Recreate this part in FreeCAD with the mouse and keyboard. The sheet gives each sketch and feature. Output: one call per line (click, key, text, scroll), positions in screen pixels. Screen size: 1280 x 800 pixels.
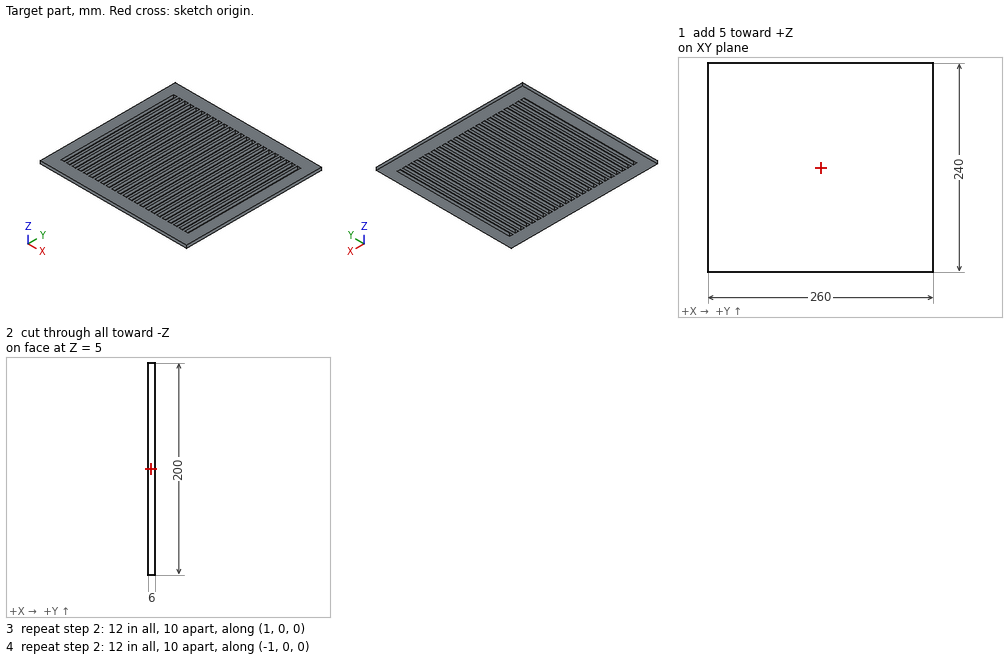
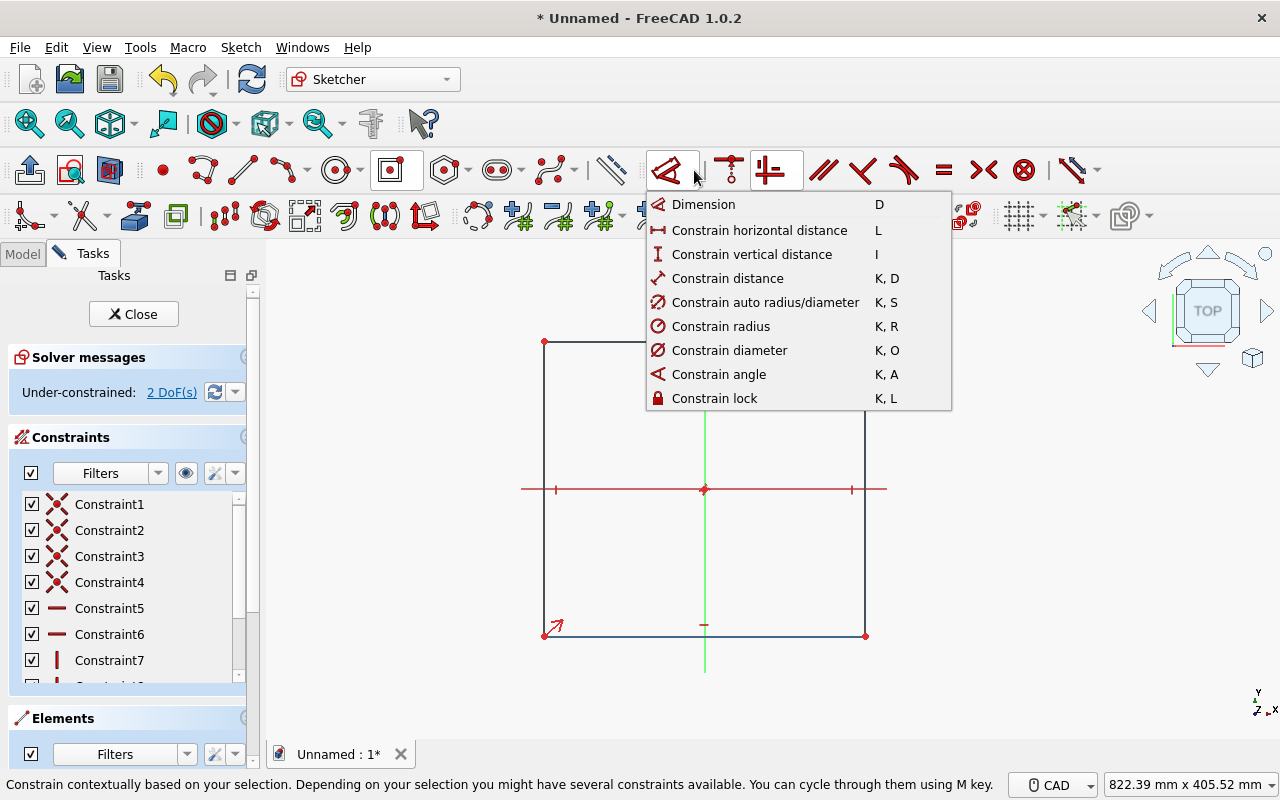
click(799, 230)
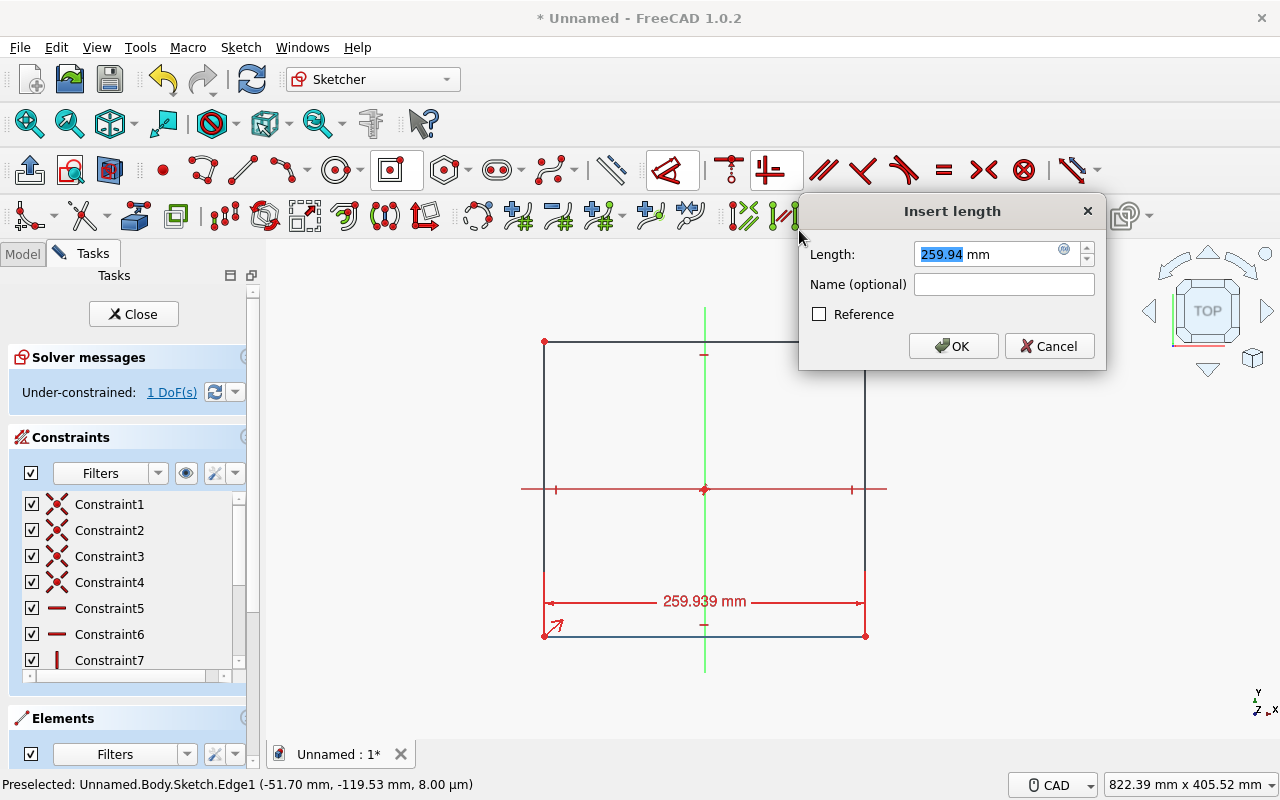
text(260)
key(Return)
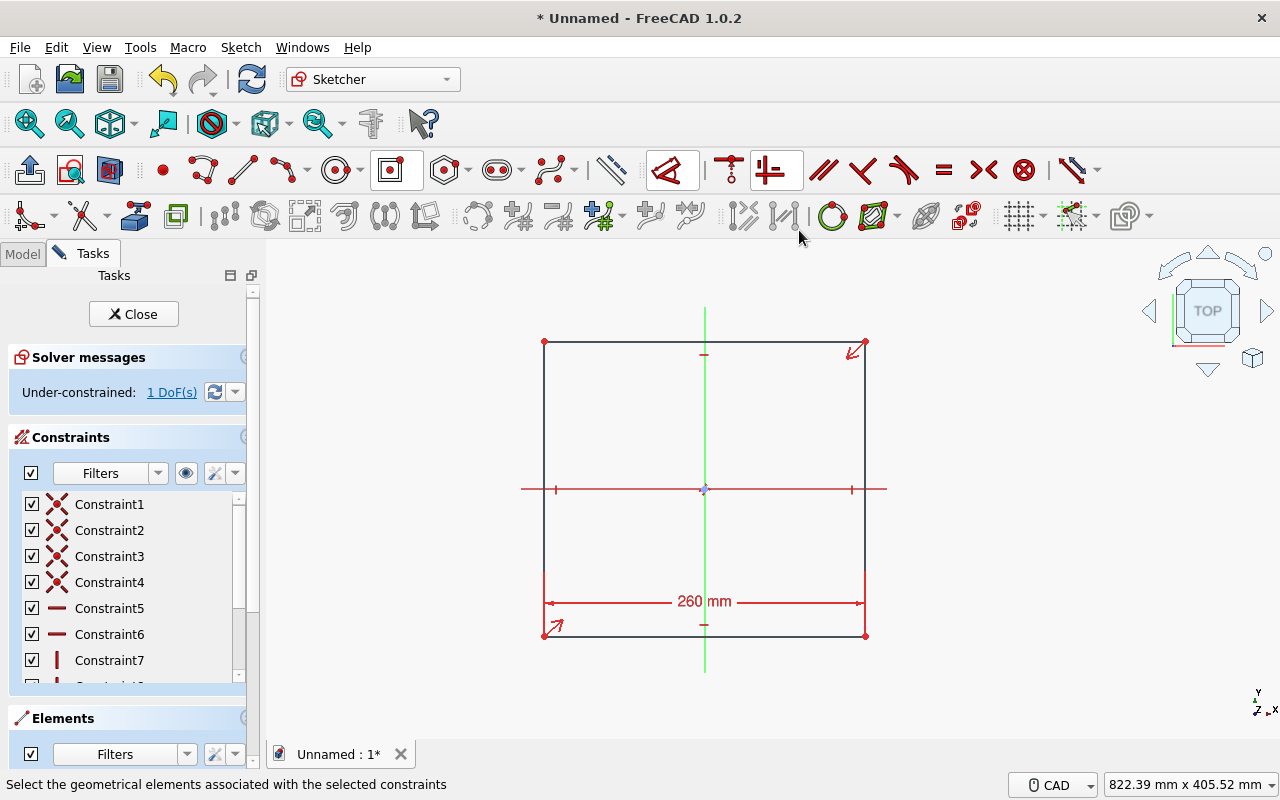
click(865, 548)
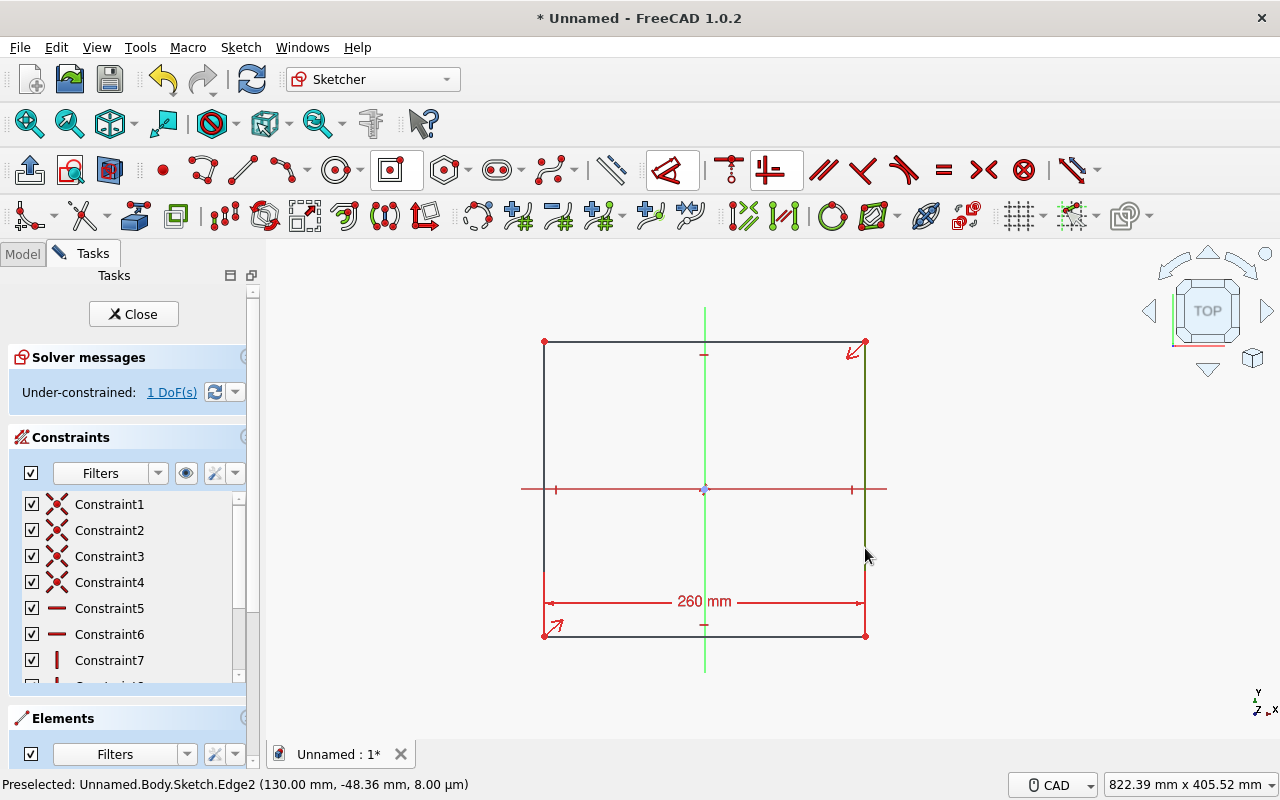
click(694, 170)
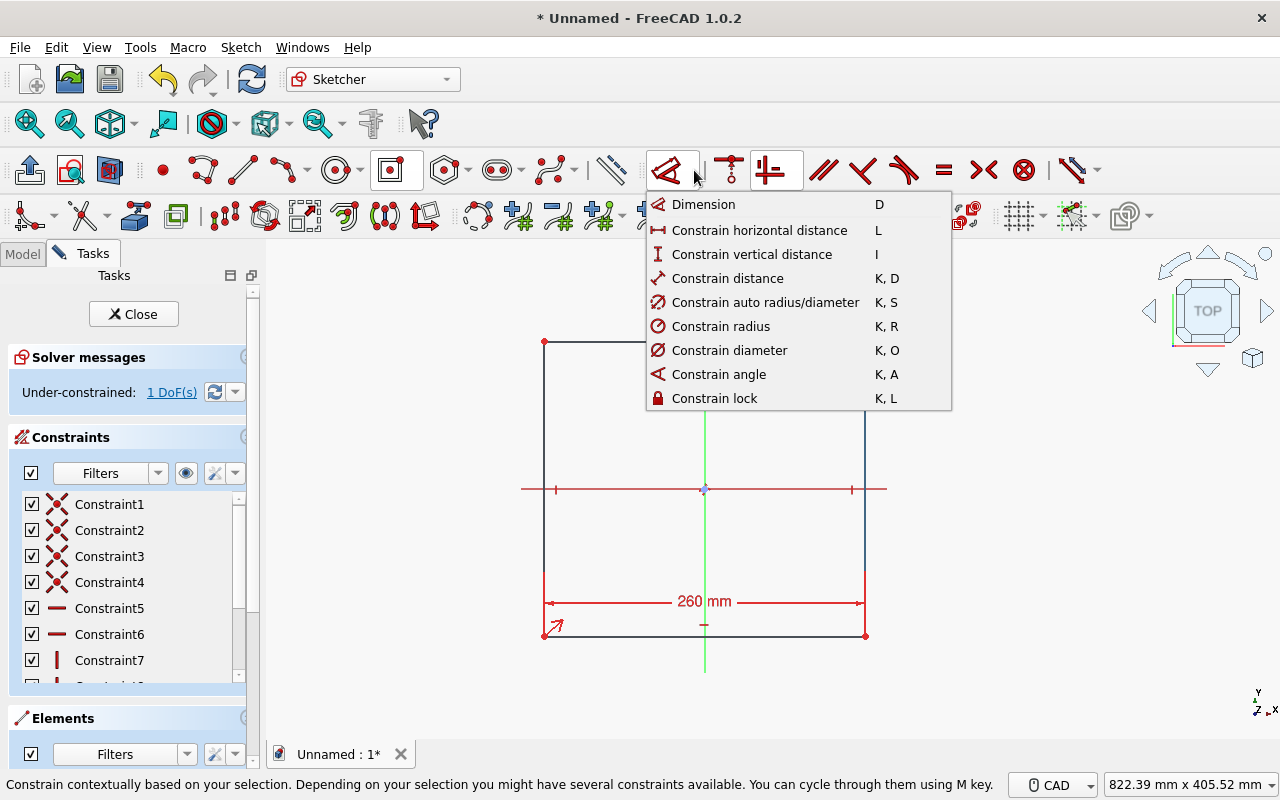
click(799, 254)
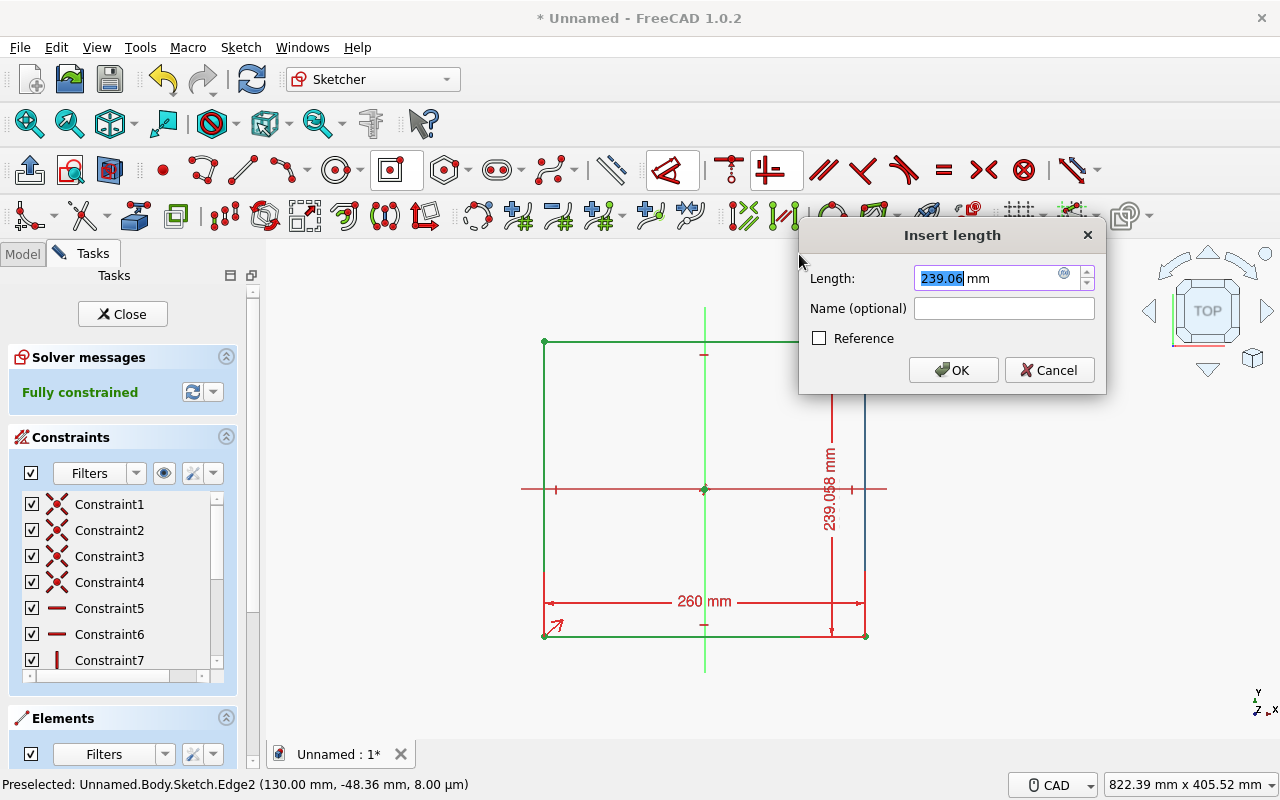
text(240)
key(Return)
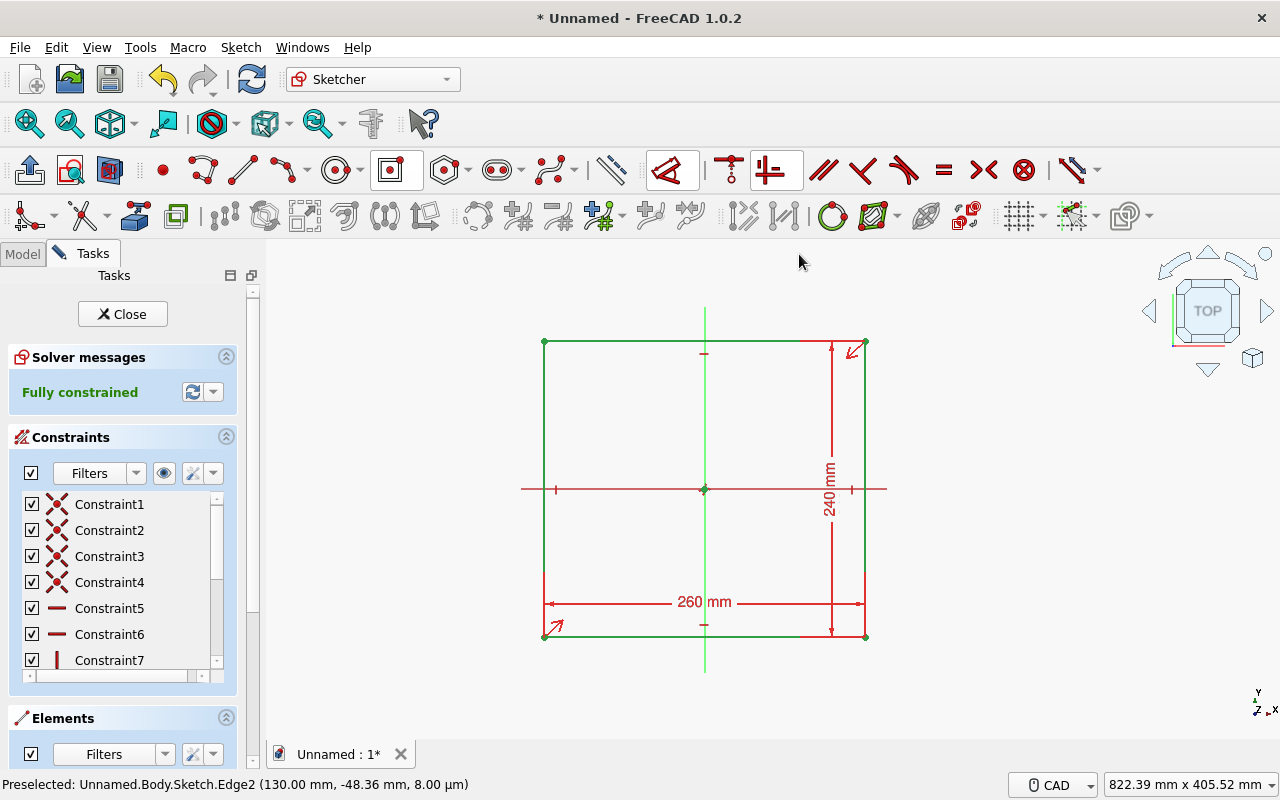
click(123, 314)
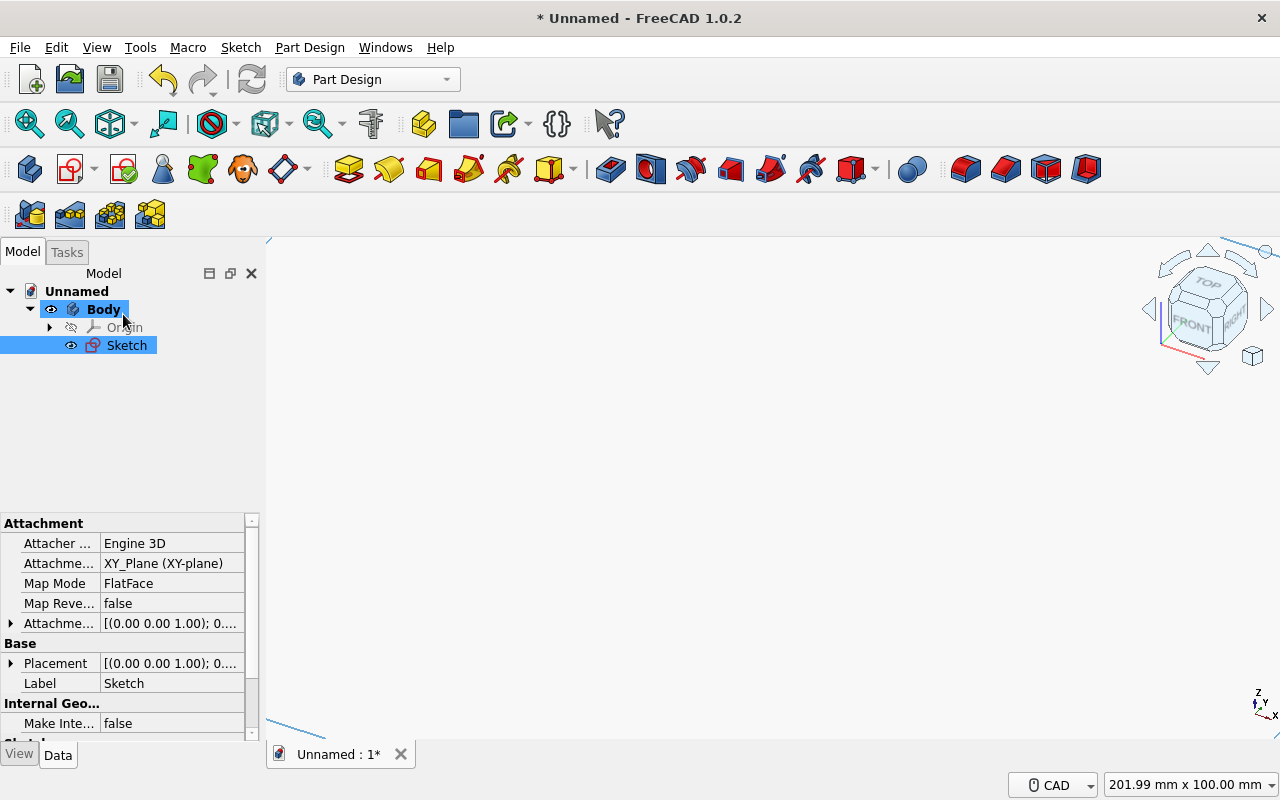
click(350, 170)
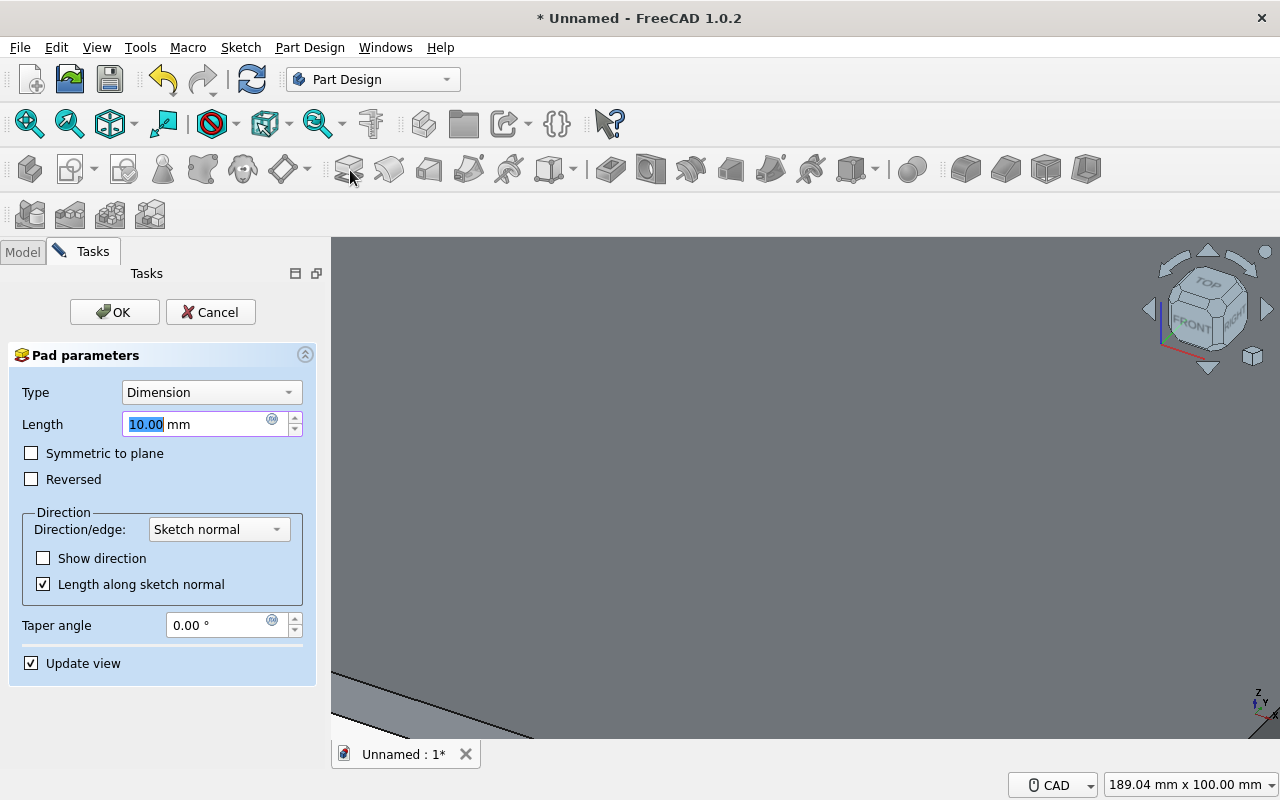
text(5)
key(Tab)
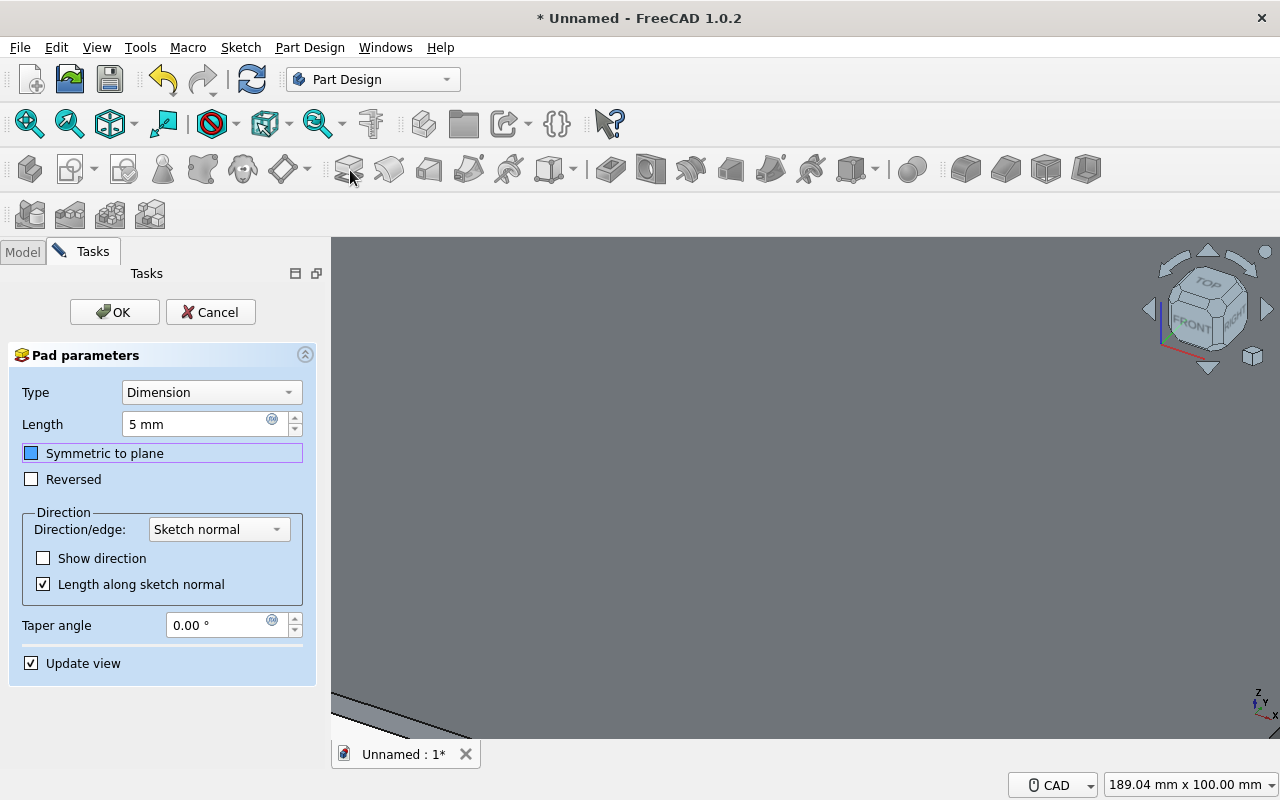
click(115, 312)